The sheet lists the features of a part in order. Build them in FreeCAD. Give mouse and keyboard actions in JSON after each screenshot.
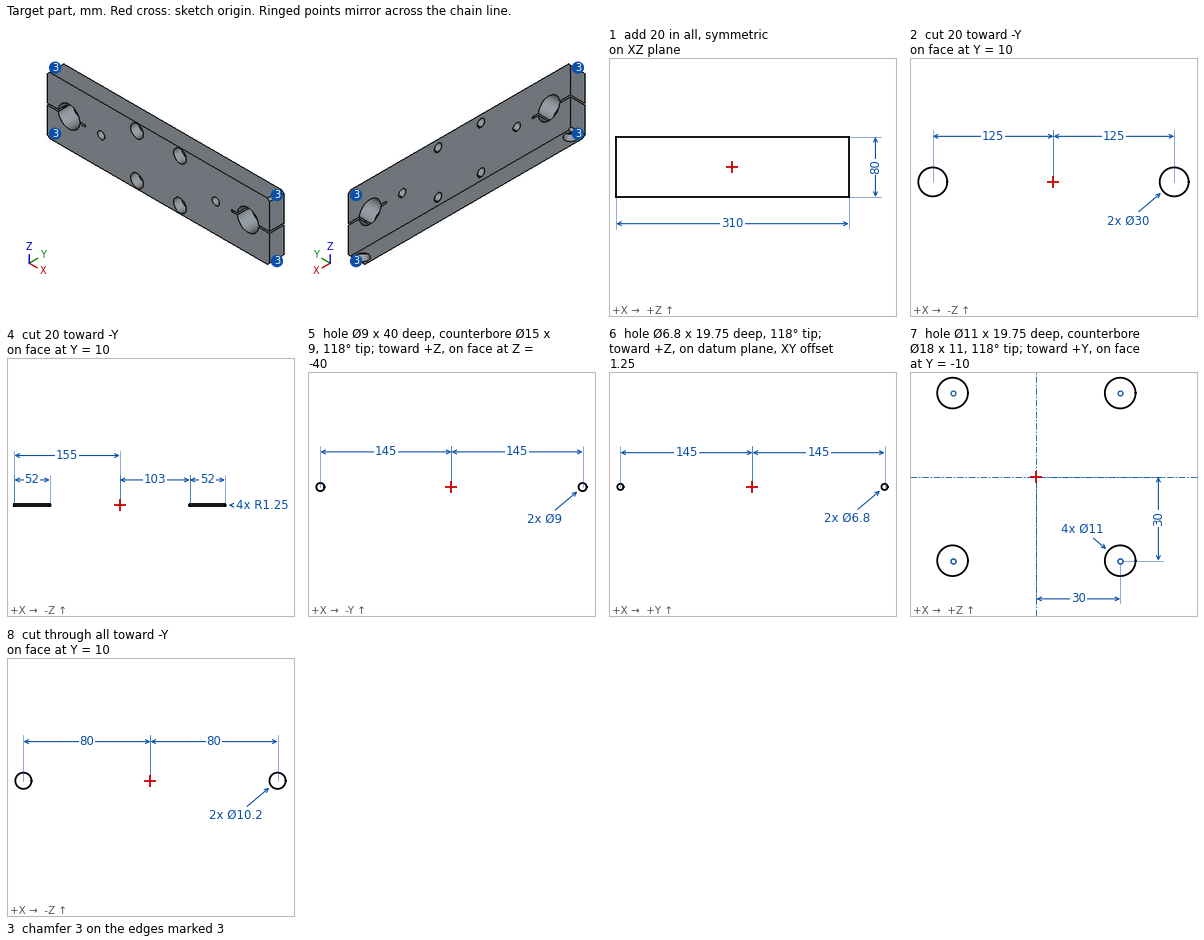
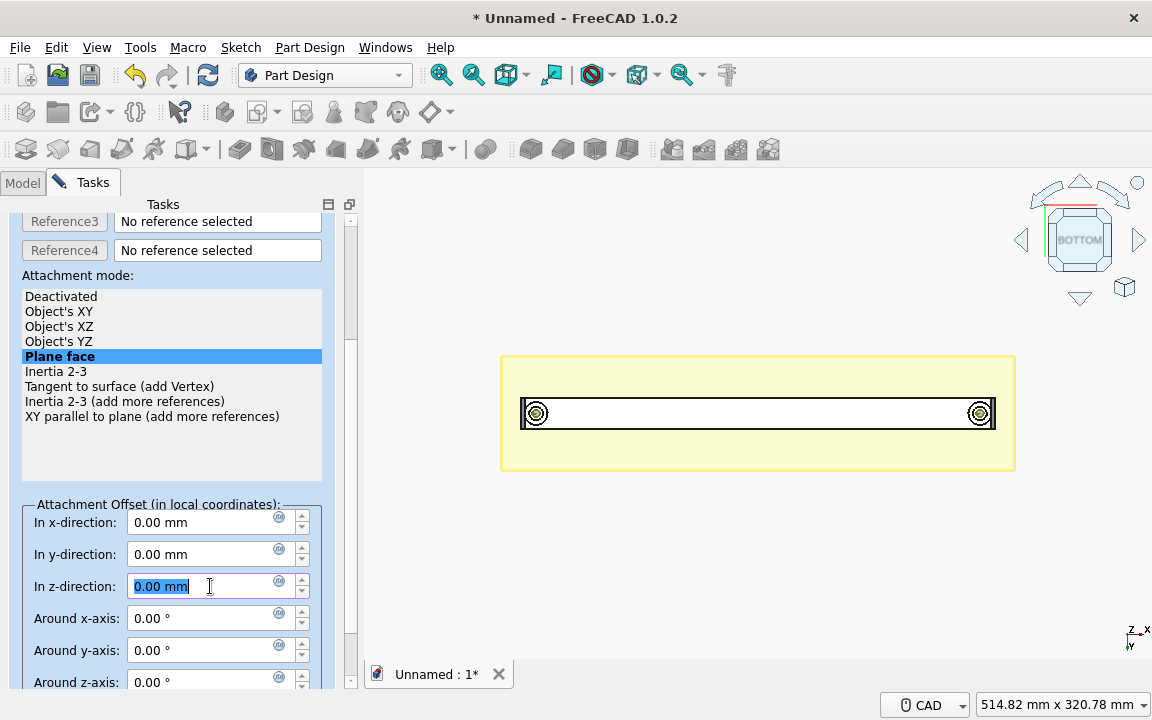
{"action": "type", "text": "1.25"}
{"action": "key", "text": "Tab"}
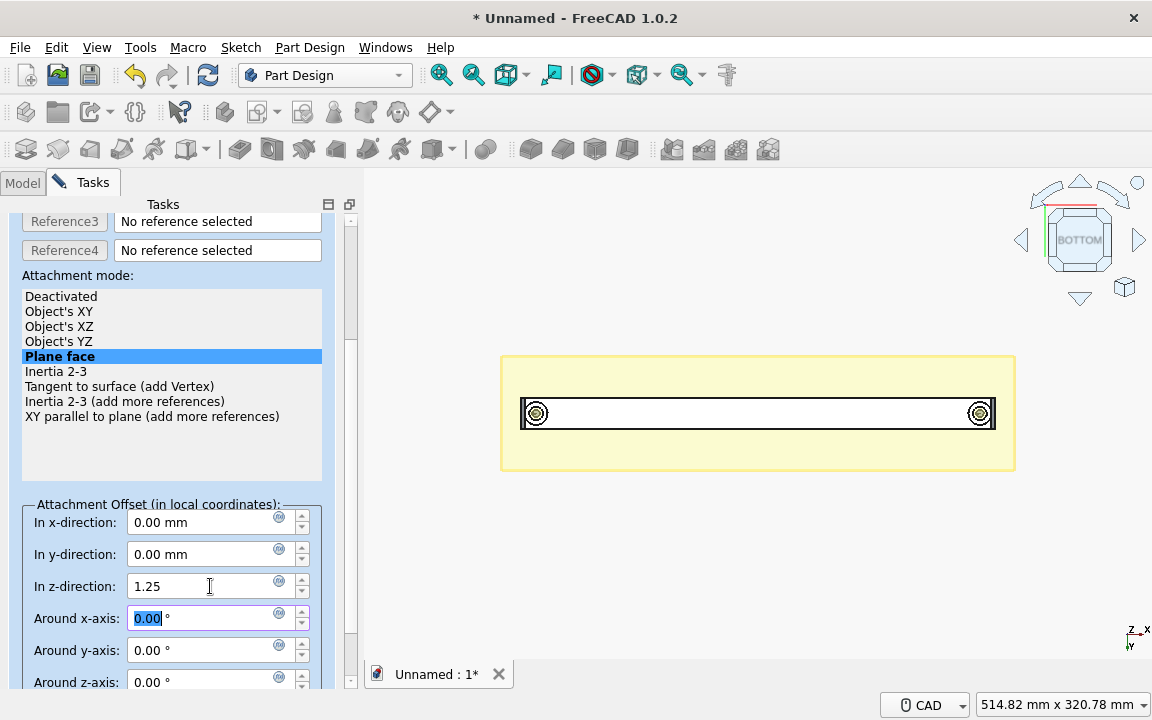
{"action": "scroll", "coordinate": [351, 451], "scroll_direction": "up", "scroll_amount": 4}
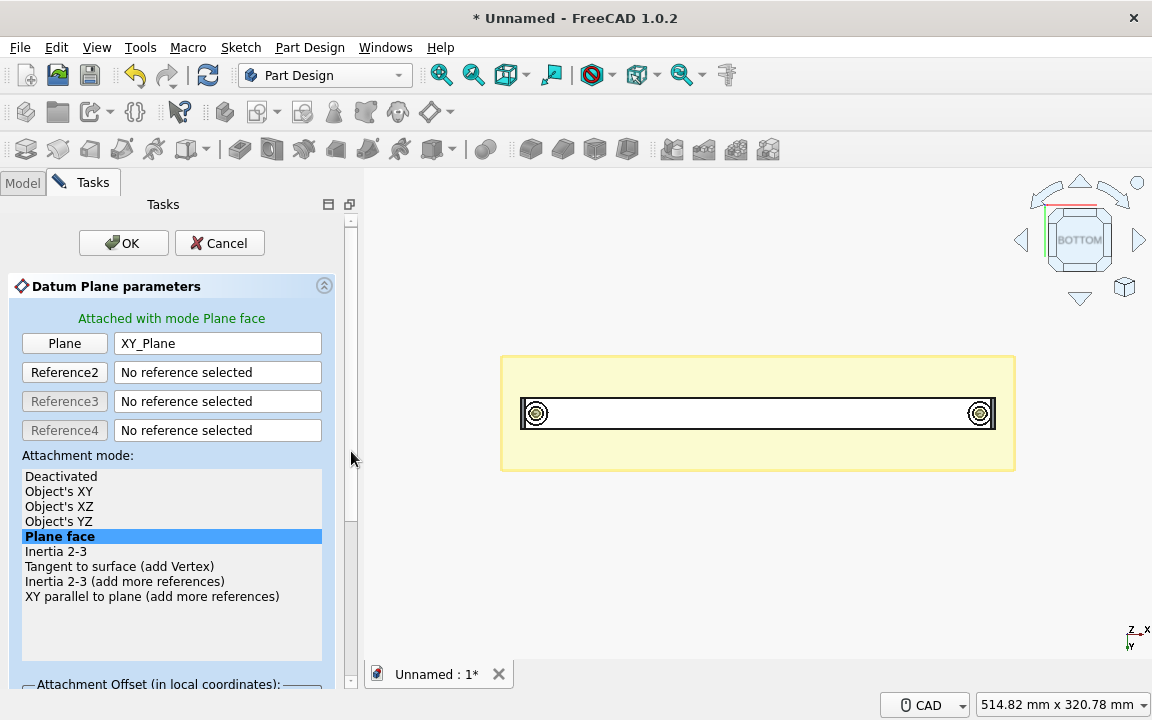
{"action": "left_click", "coordinate": [124, 243]}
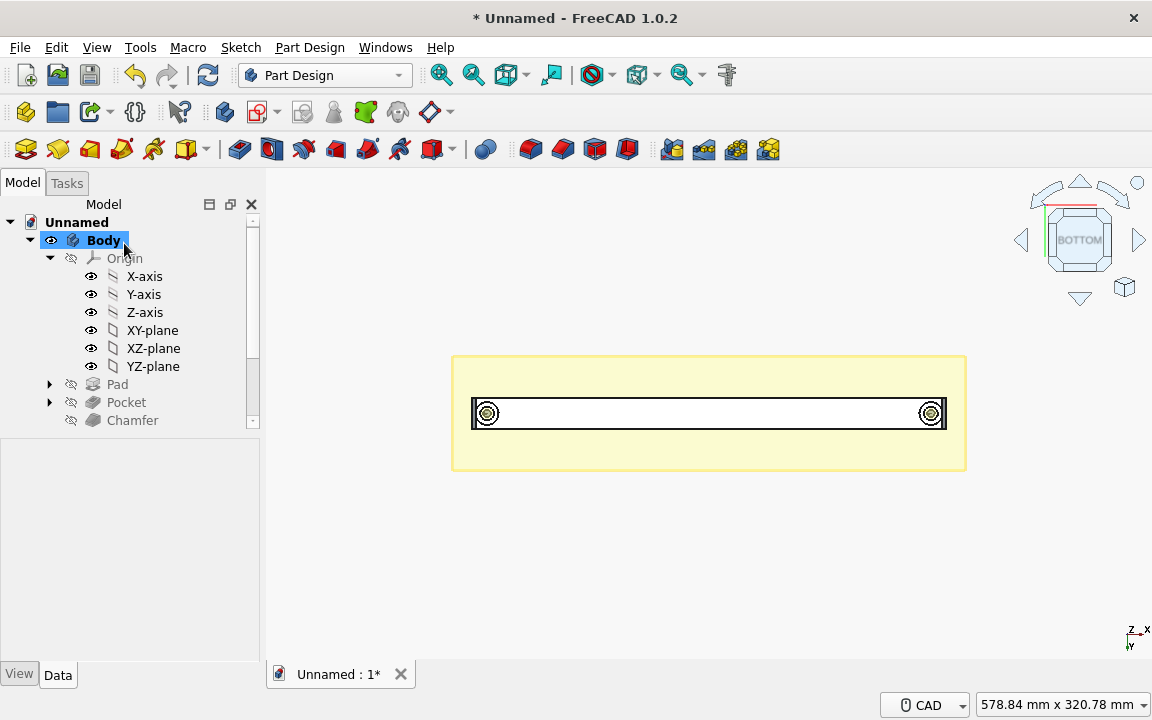
{"action": "scroll", "coordinate": [100, 326], "scroll_direction": "down", "scroll_amount": 3}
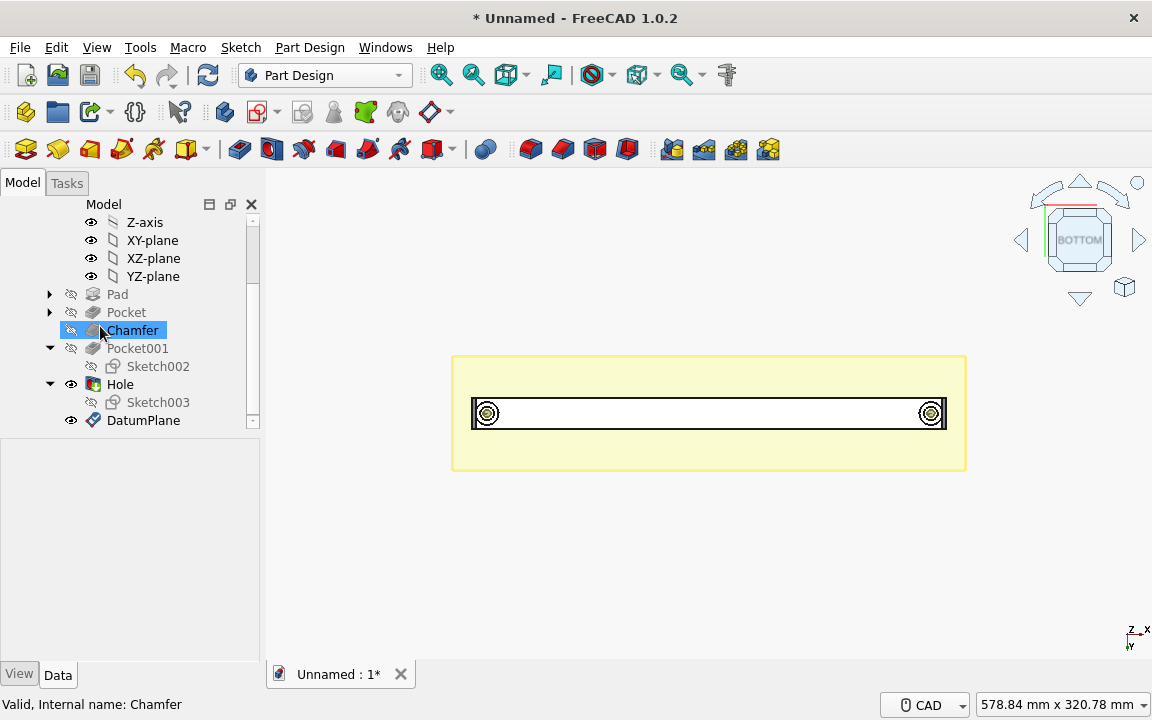
{"action": "left_click", "coordinate": [116, 420]}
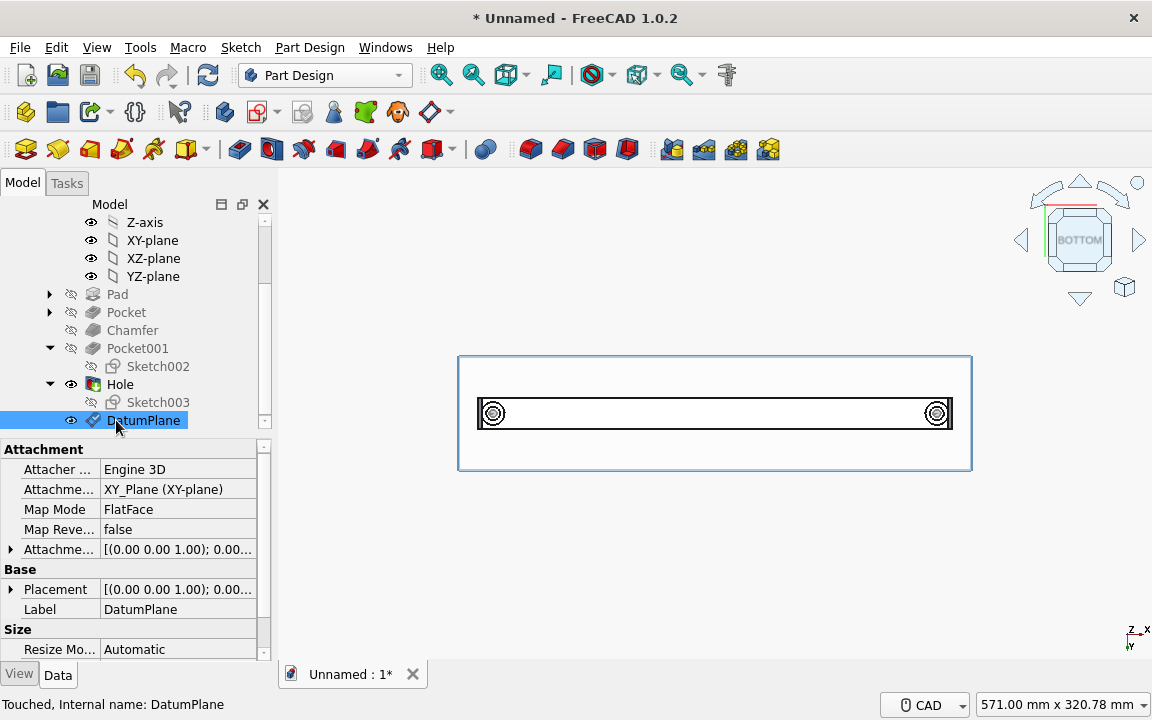
{"action": "left_click", "coordinate": [258, 112]}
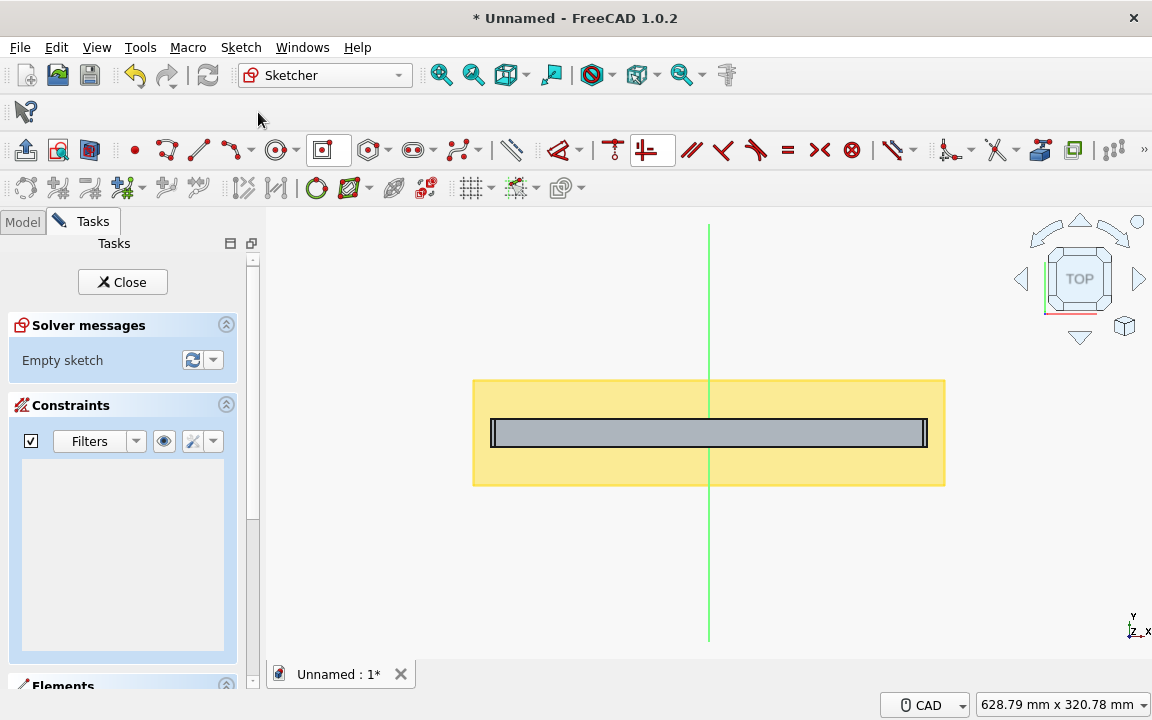
{"action": "left_click", "coordinate": [90, 150]}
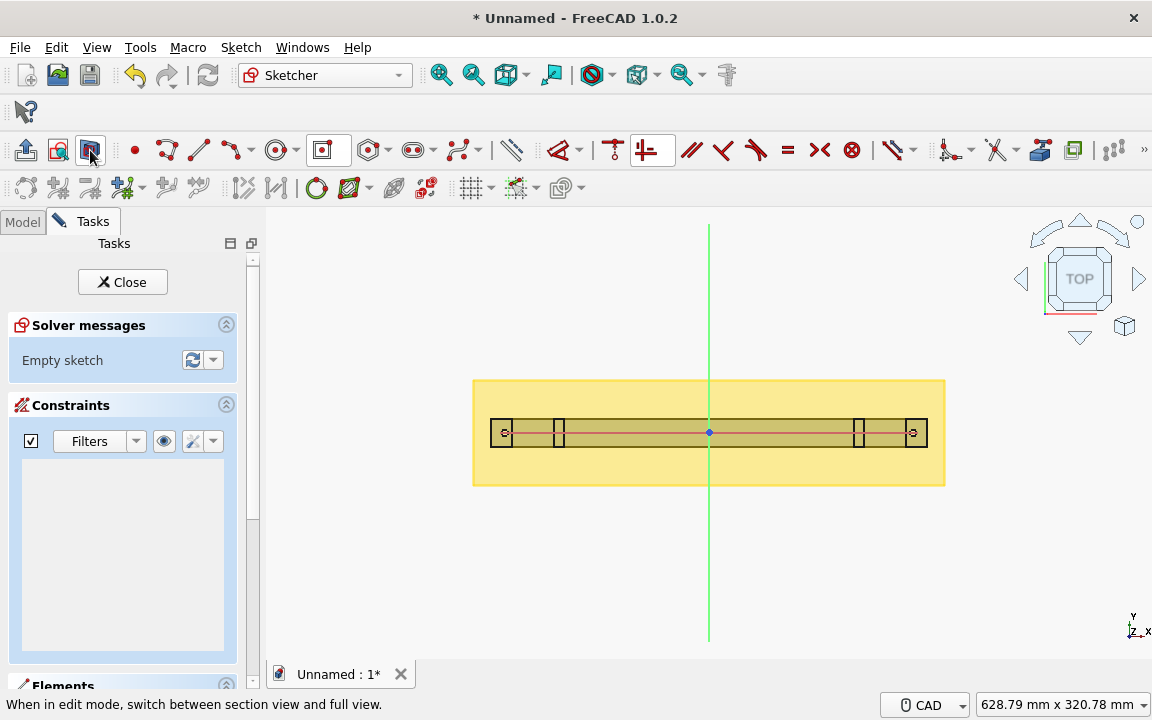
{"action": "left_click", "coordinate": [276, 150]}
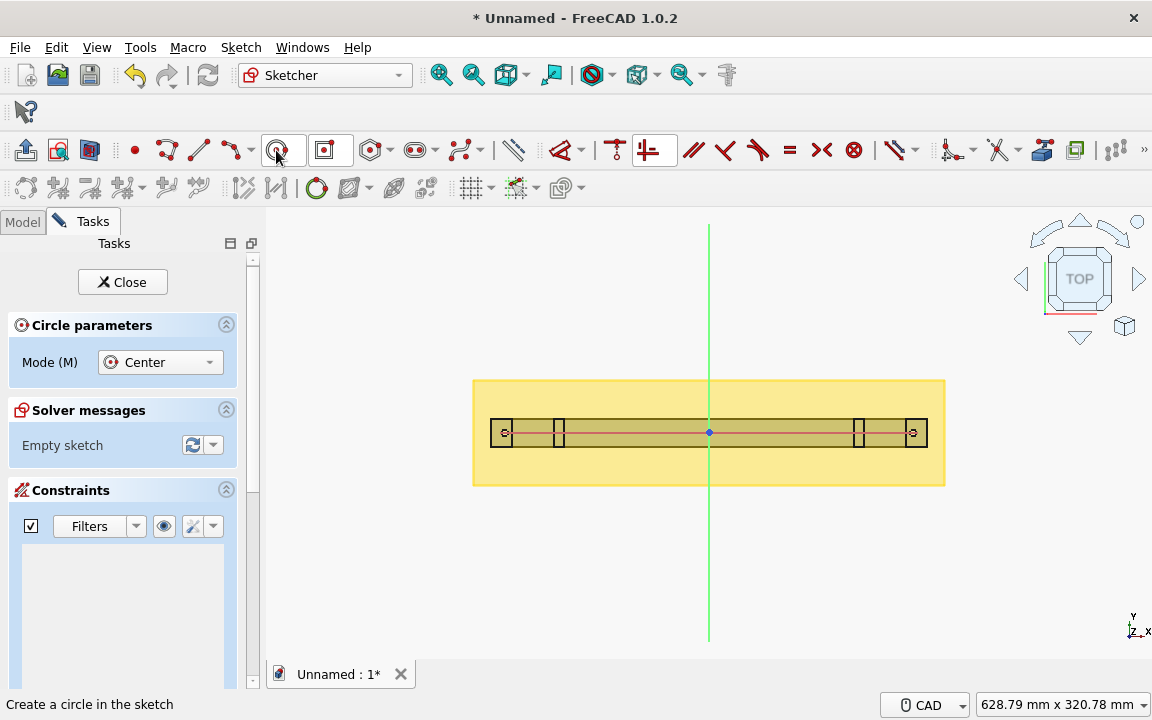
{"action": "scroll", "coordinate": [913, 433], "scroll_direction": "up", "scroll_amount": 8}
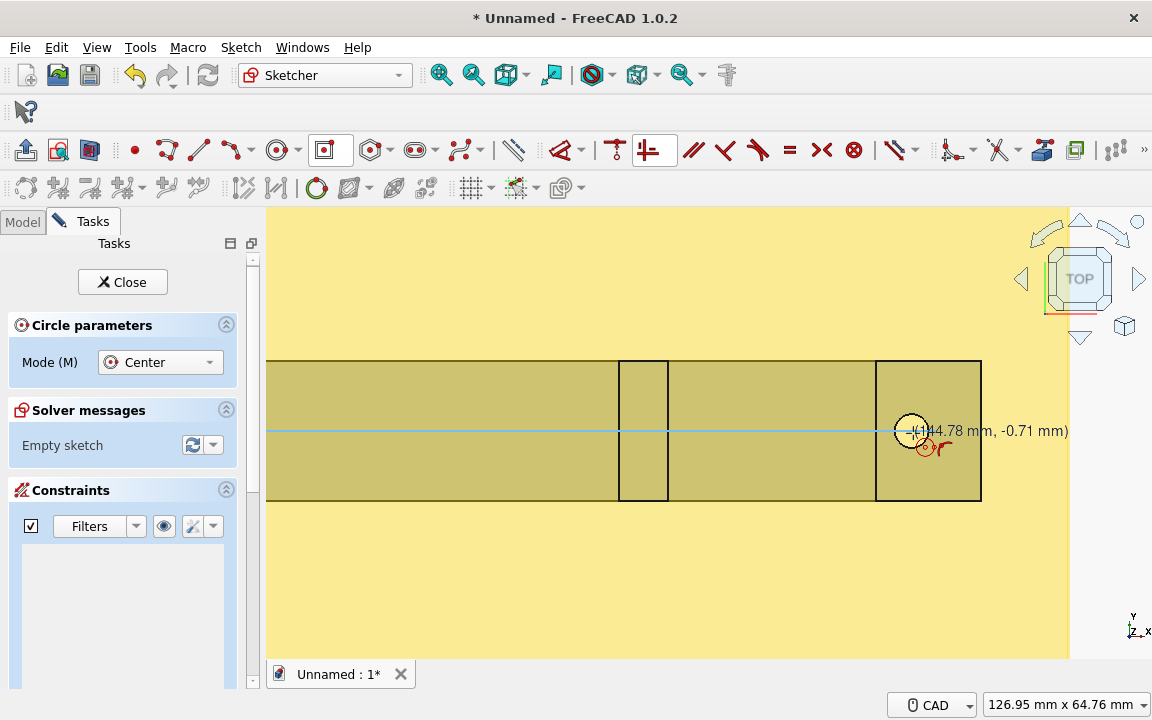
{"action": "scroll", "coordinate": [883, 434], "scroll_direction": "down", "scroll_amount": 7}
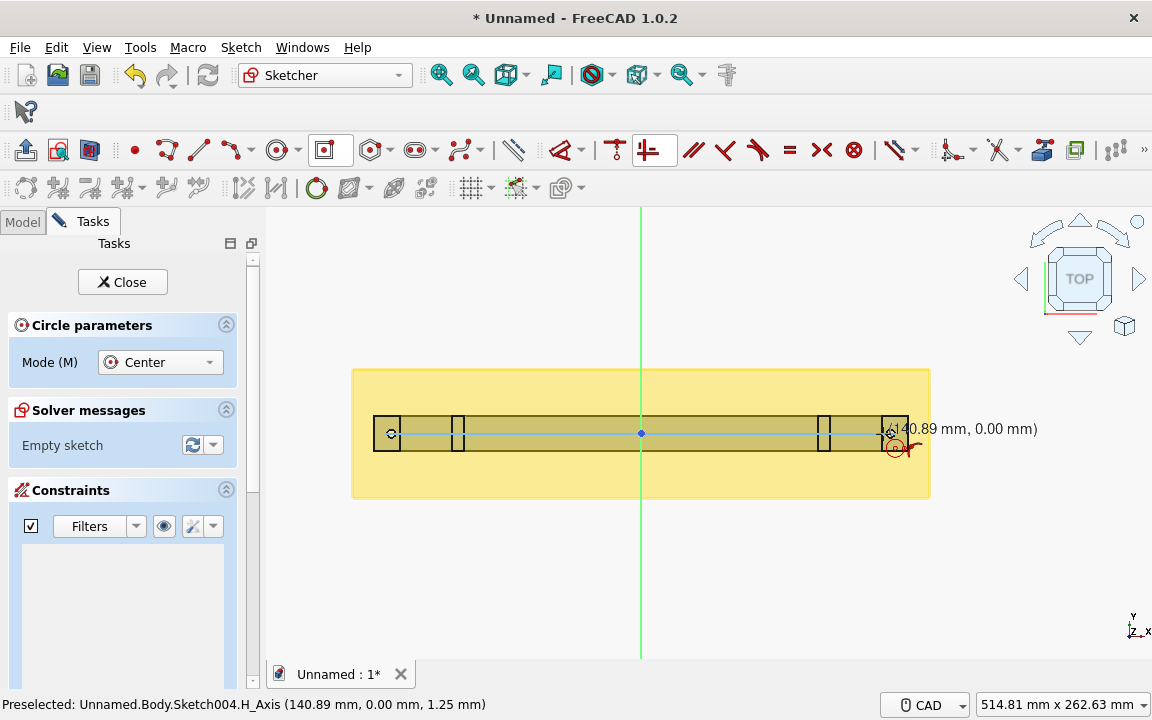
{"action": "left_click", "coordinate": [891, 434]}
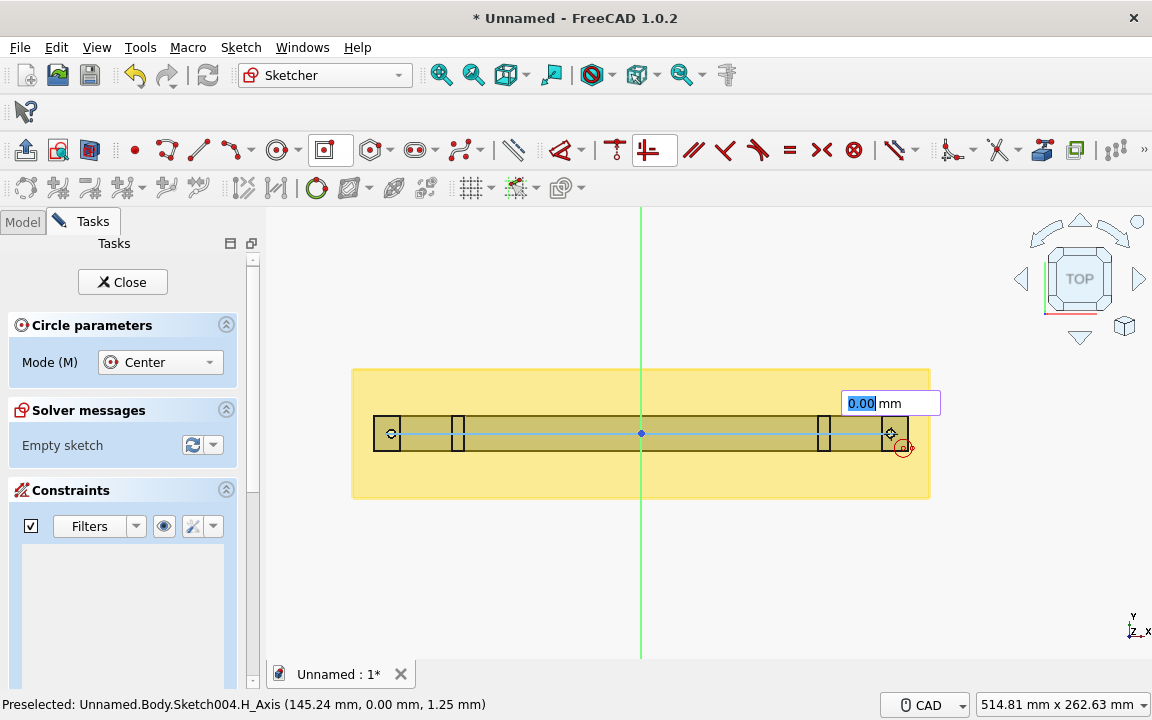
{"action": "scroll", "coordinate": [889, 439], "scroll_direction": "up", "scroll_amount": 6}
{"action": "mouse_move", "coordinate": [886, 438]}